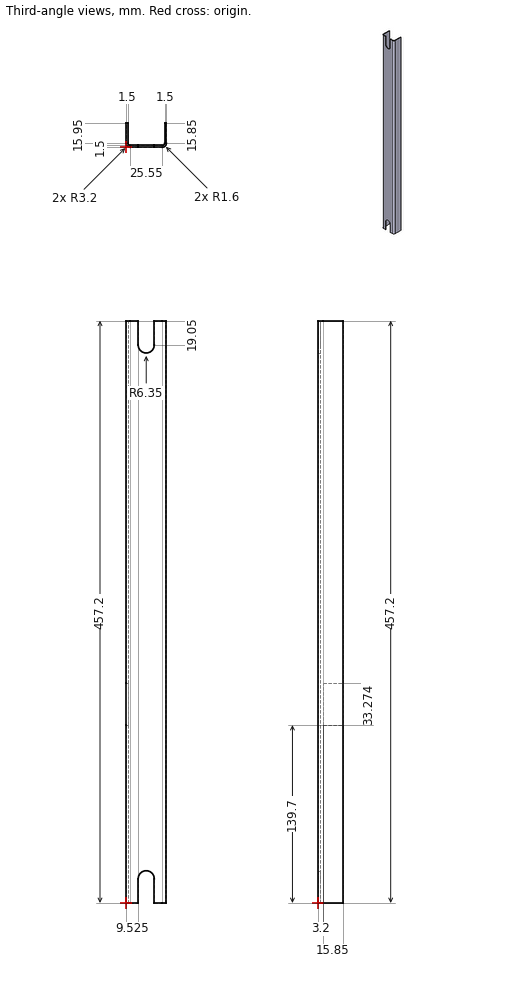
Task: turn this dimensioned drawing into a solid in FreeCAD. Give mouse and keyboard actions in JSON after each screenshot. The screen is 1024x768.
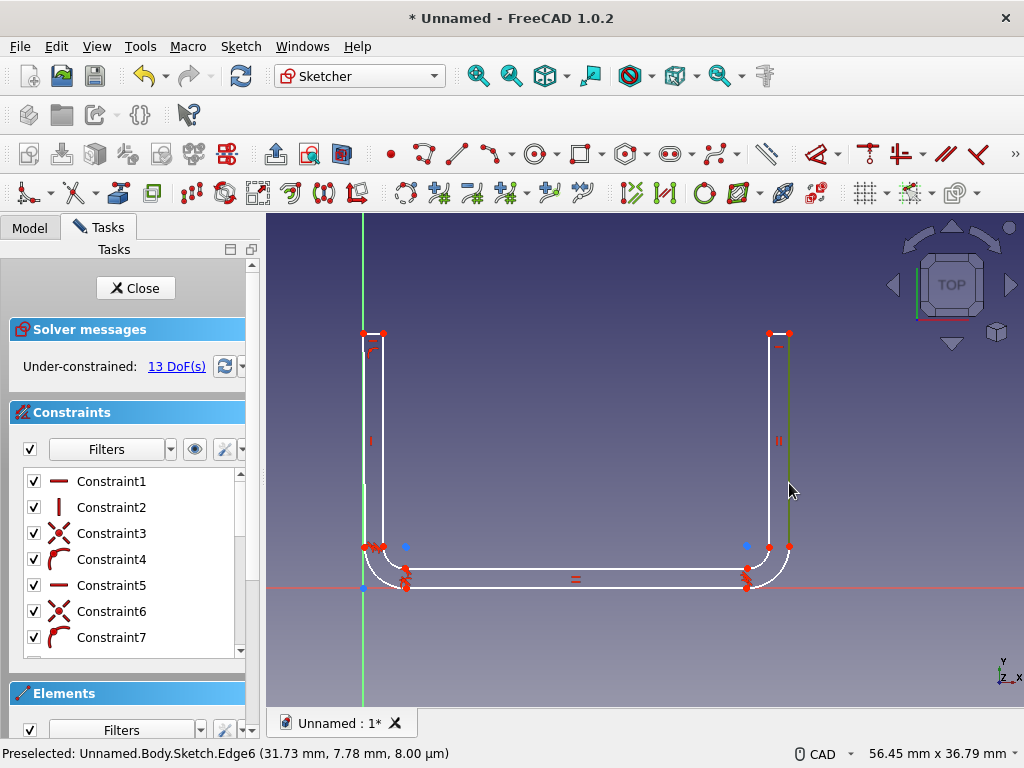
{"action": "left_click", "coordinate": [784, 566]}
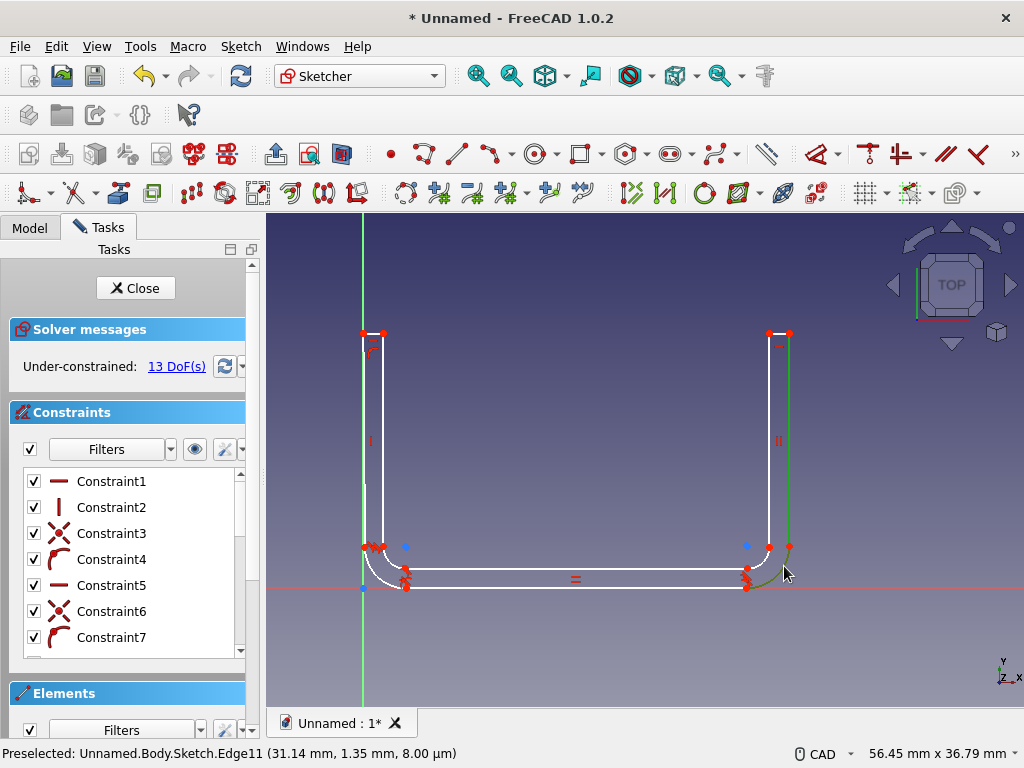
{"action": "key", "text": "t"}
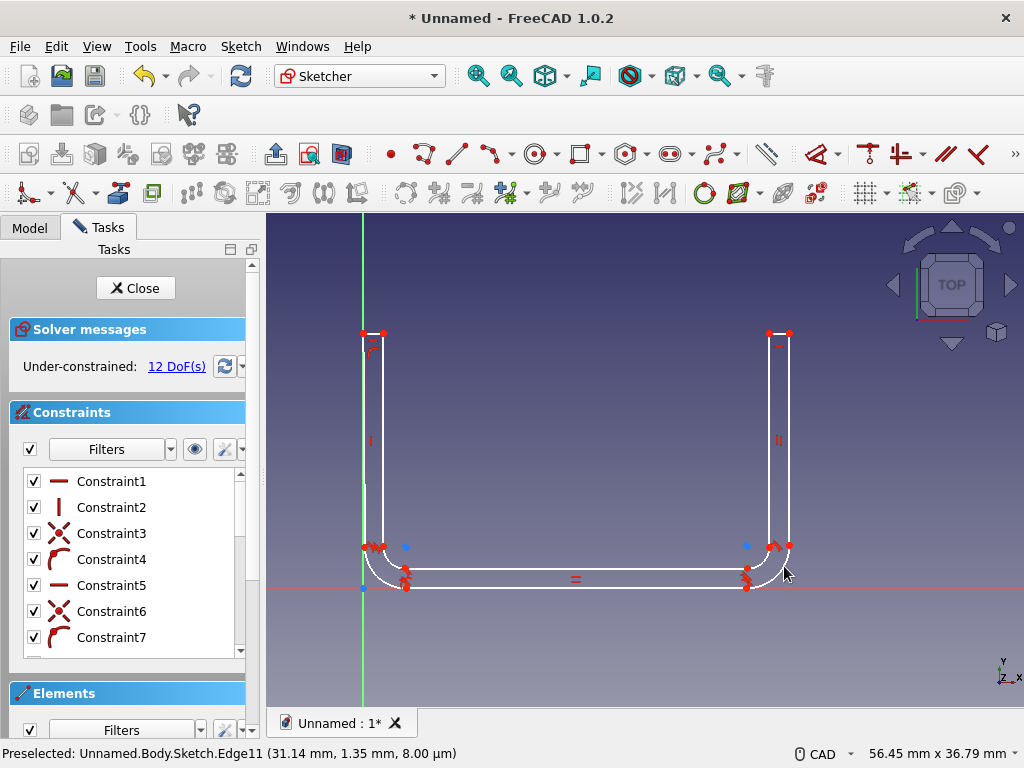
{"action": "left_click", "coordinate": [769, 398]}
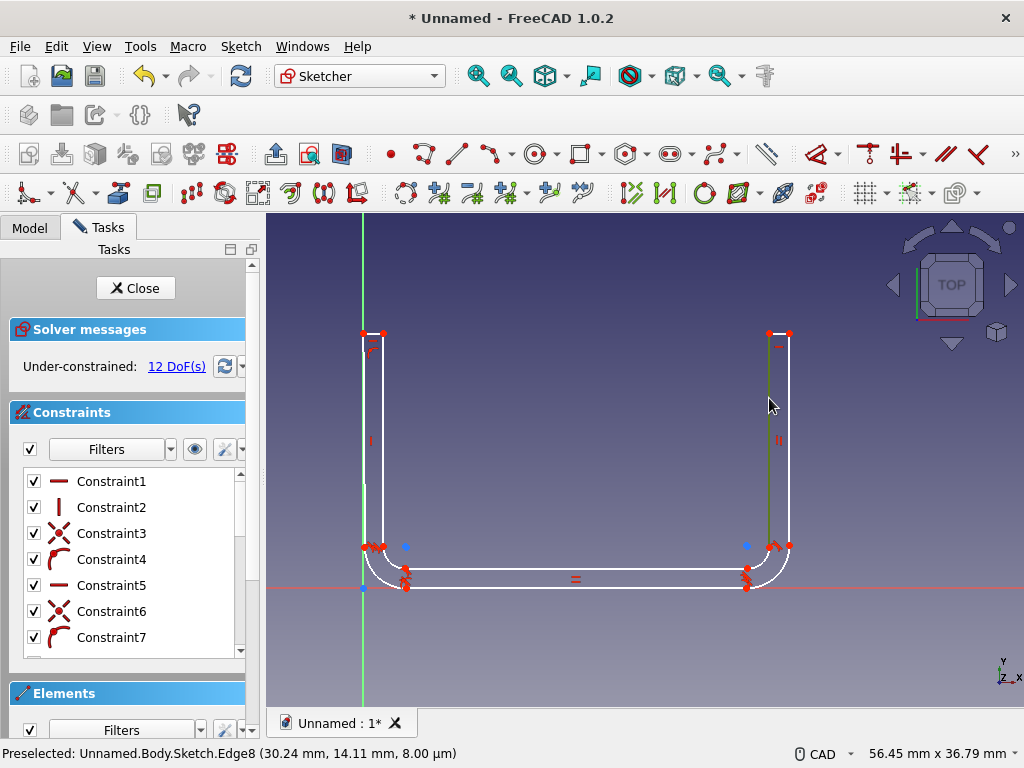
{"action": "scroll", "coordinate": [757, 567], "scroll_direction": "up", "scroll_amount": 2}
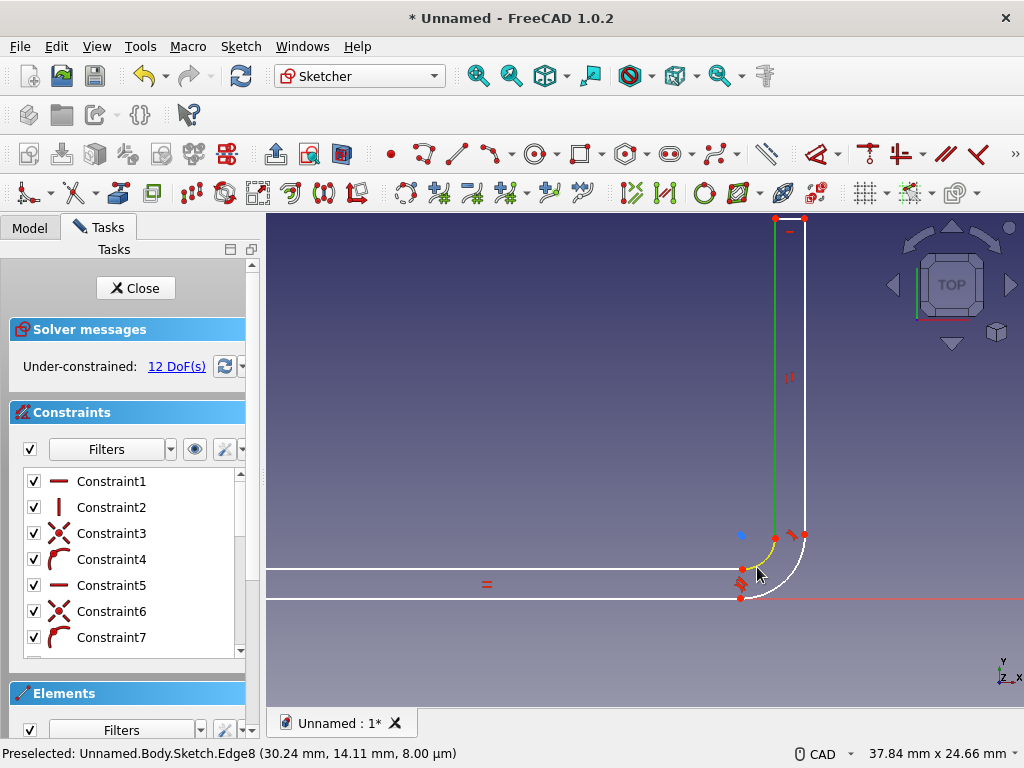
{"action": "left_click", "coordinate": [757, 566]}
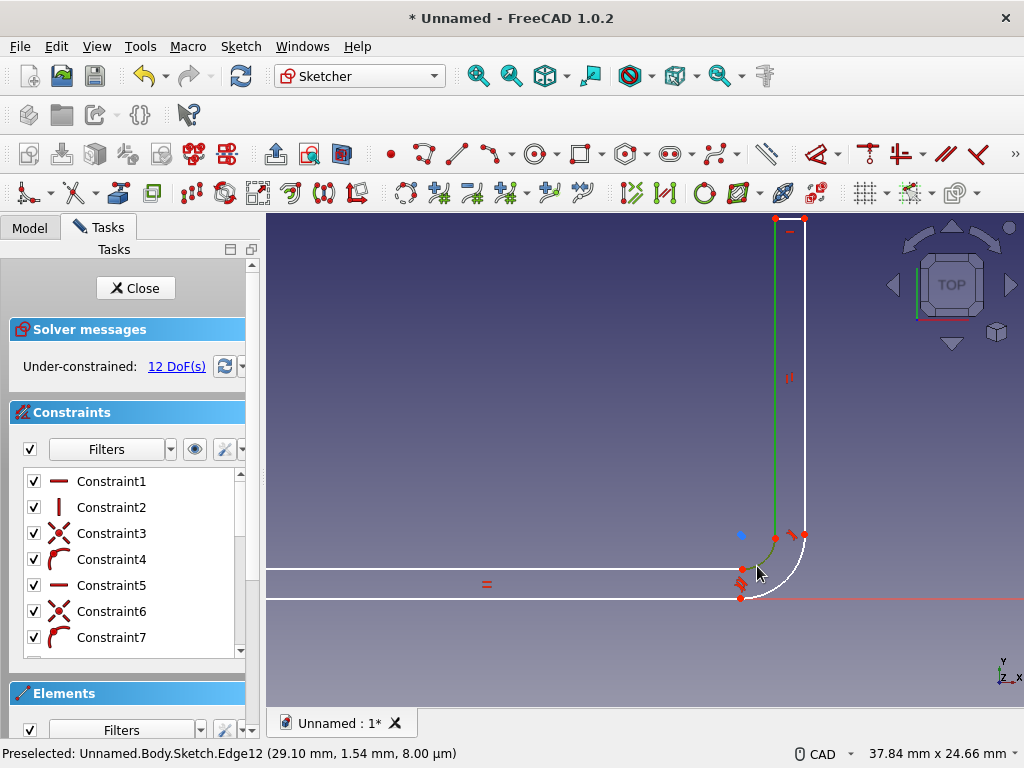
{"action": "key", "text": "t"}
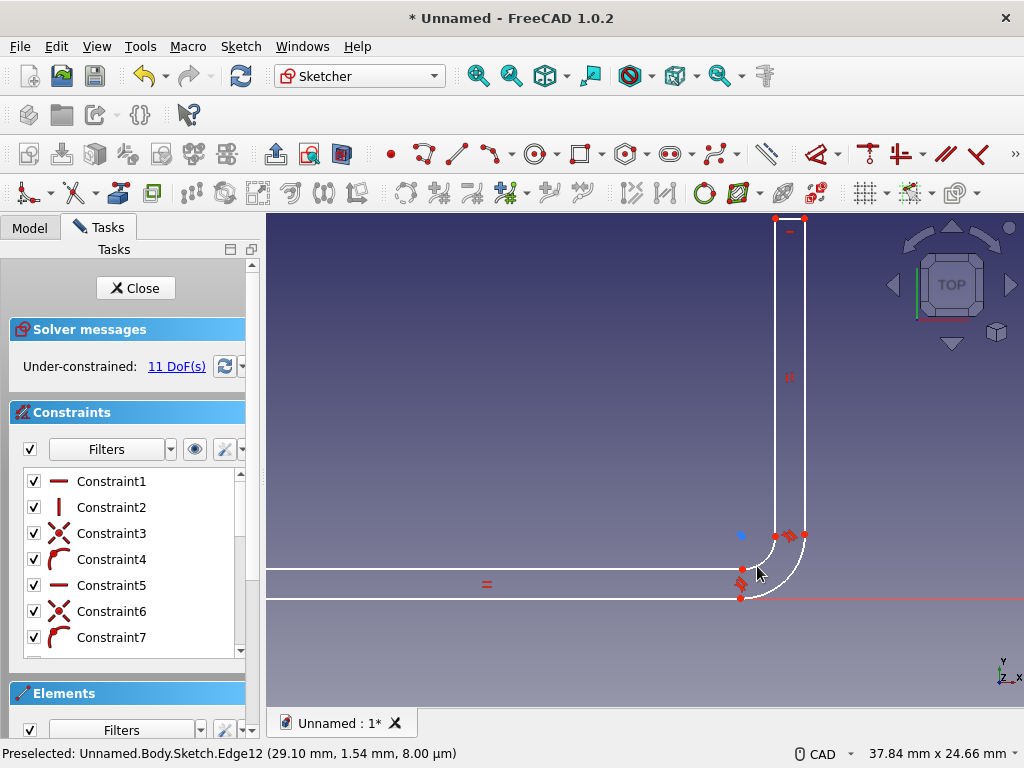
{"action": "scroll", "coordinate": [758, 566], "scroll_direction": "down", "scroll_amount": 2}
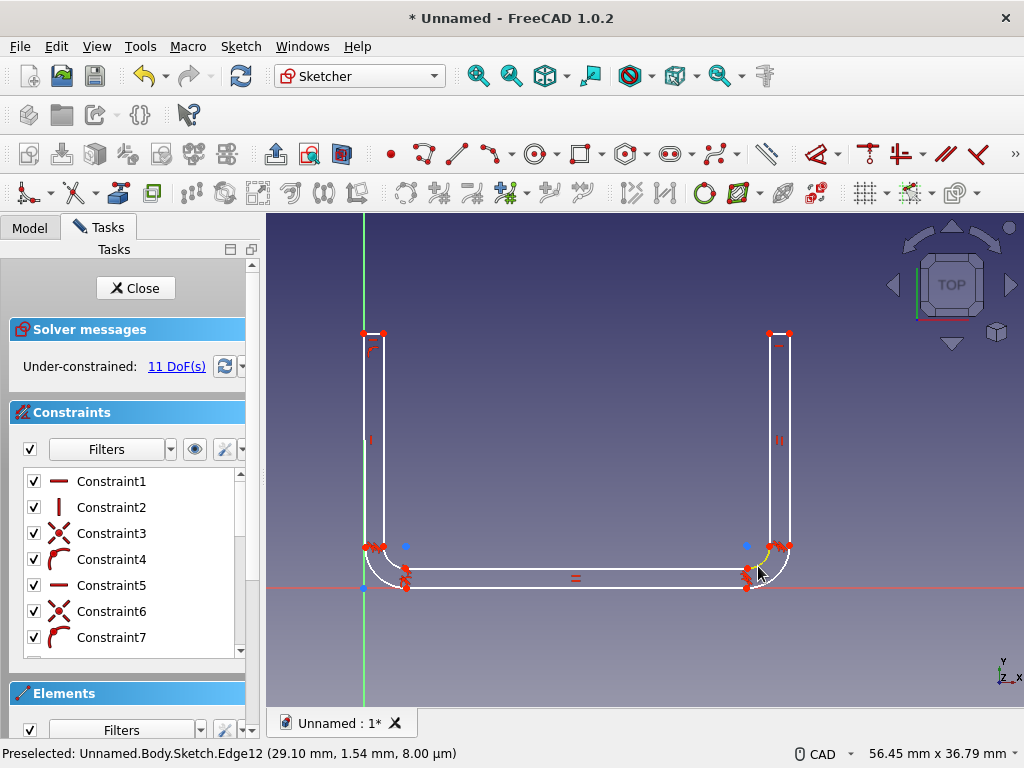
{"action": "left_click", "coordinate": [364, 398]}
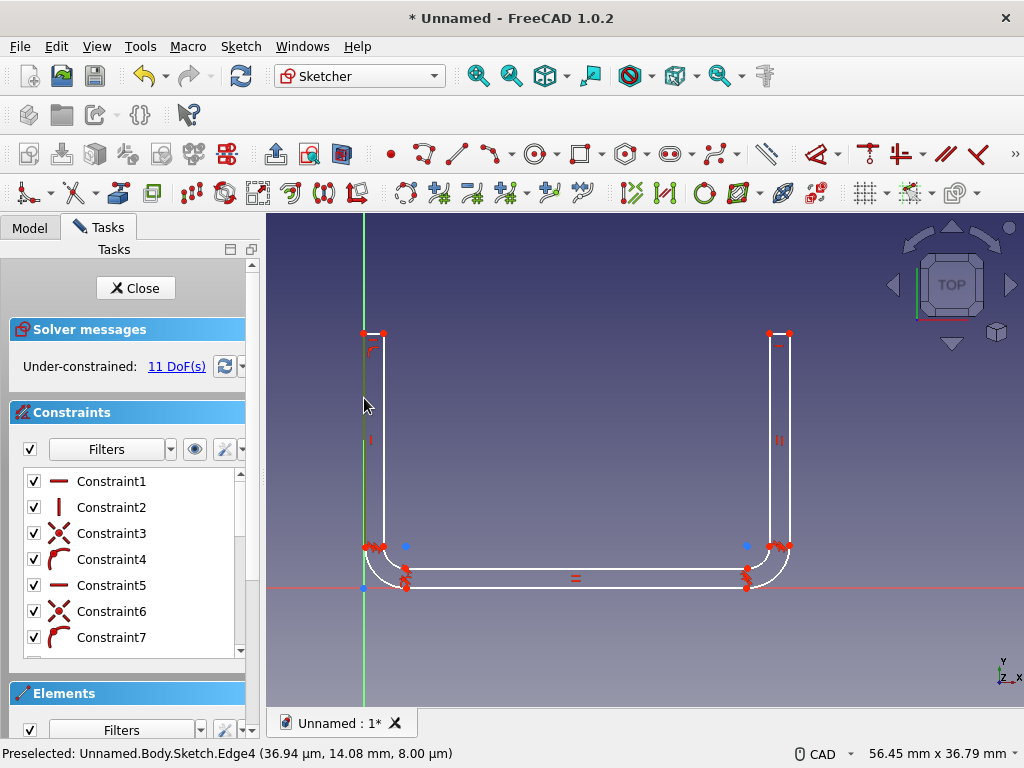
{"action": "key", "text": "v"}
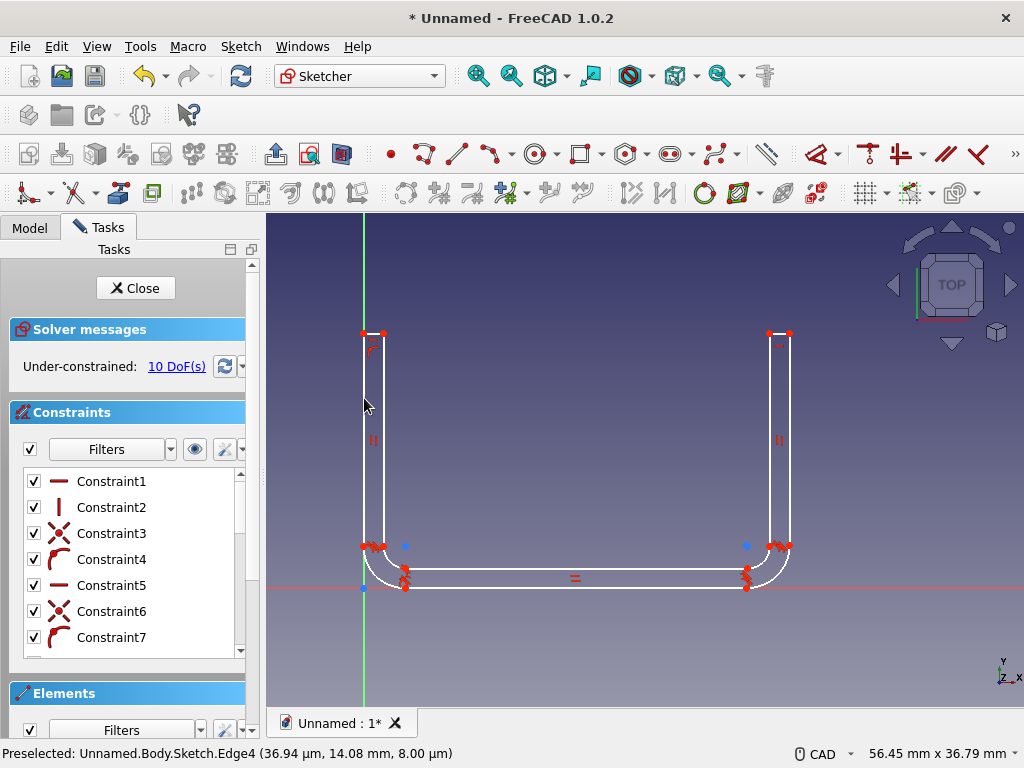
{"action": "left_click", "coordinate": [376, 576]}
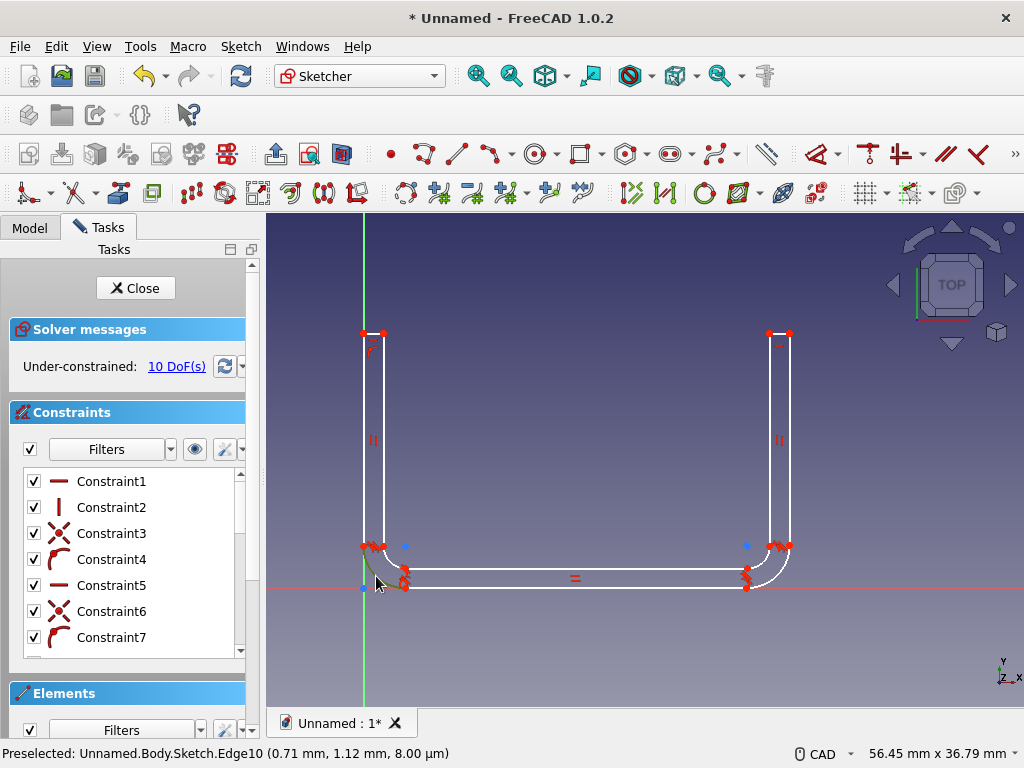
{"action": "left_click", "coordinate": [785, 565]}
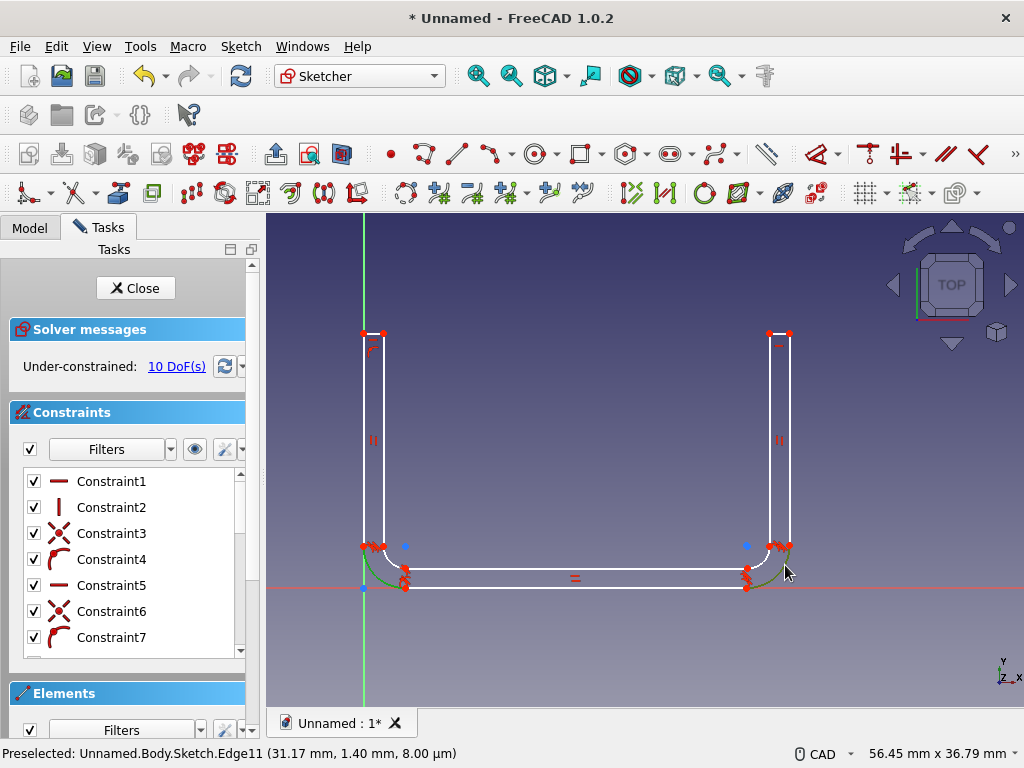
{"action": "key", "text": "e"}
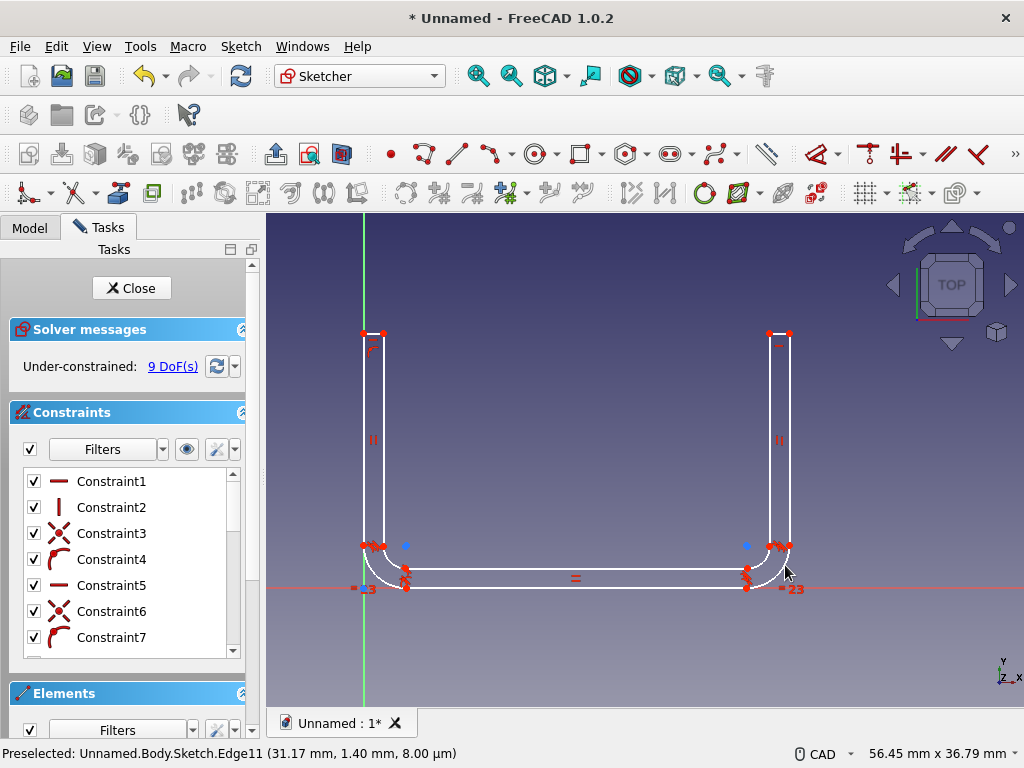
{"action": "scroll", "coordinate": [386, 556], "scroll_direction": "up", "scroll_amount": 2}